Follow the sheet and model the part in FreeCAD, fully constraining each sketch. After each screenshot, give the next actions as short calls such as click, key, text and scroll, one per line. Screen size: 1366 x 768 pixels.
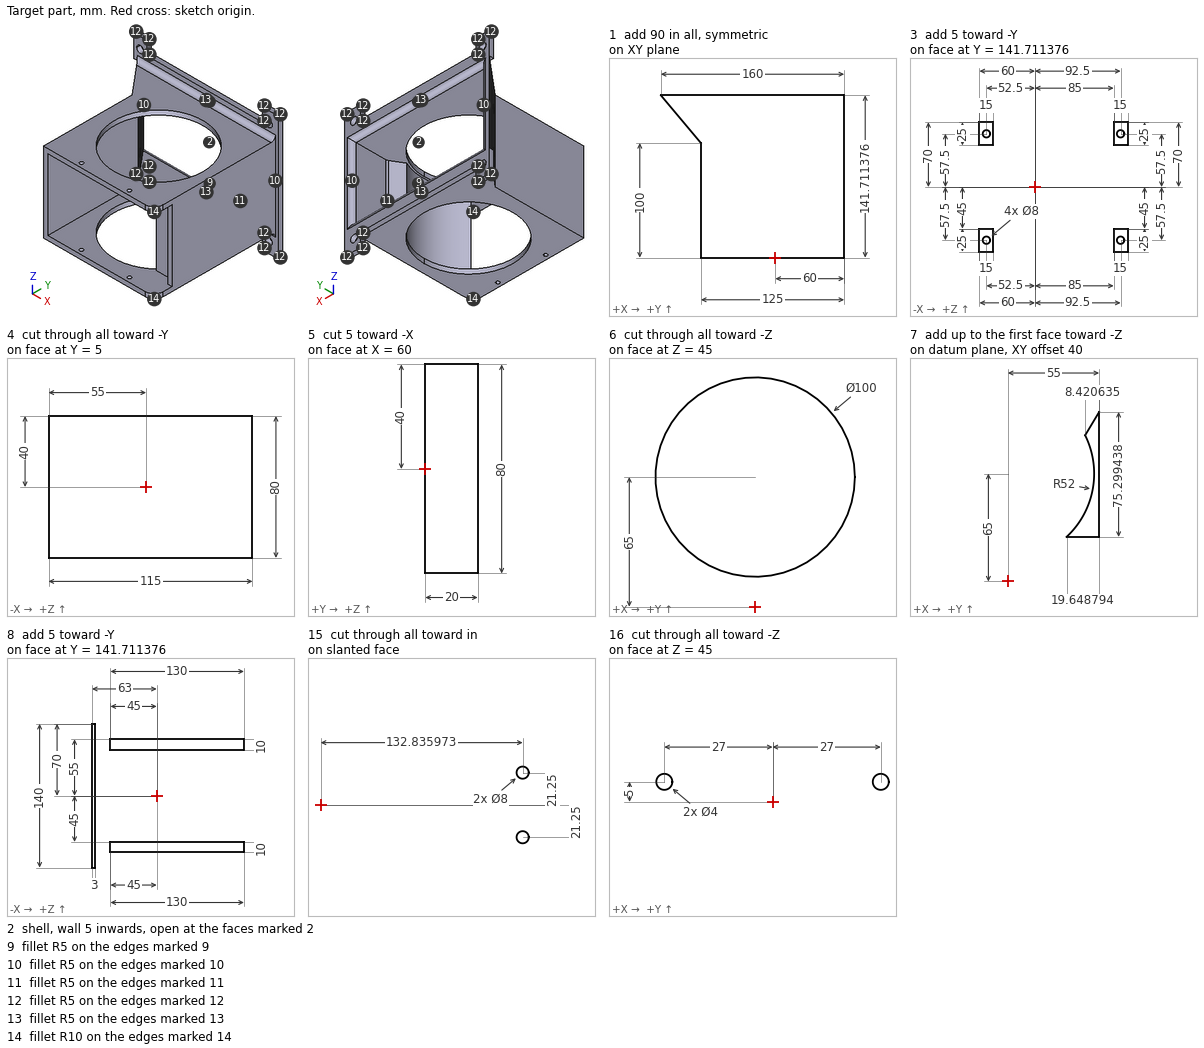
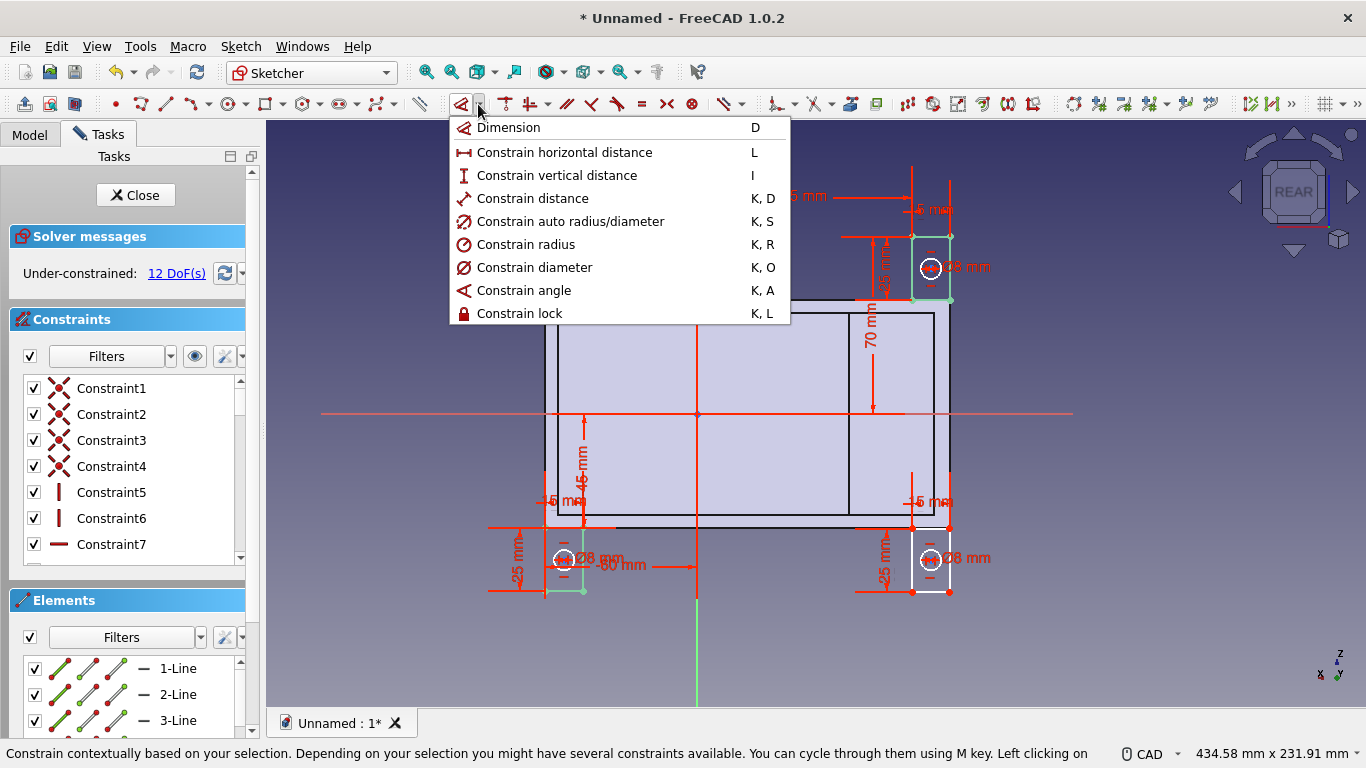
click(620, 152)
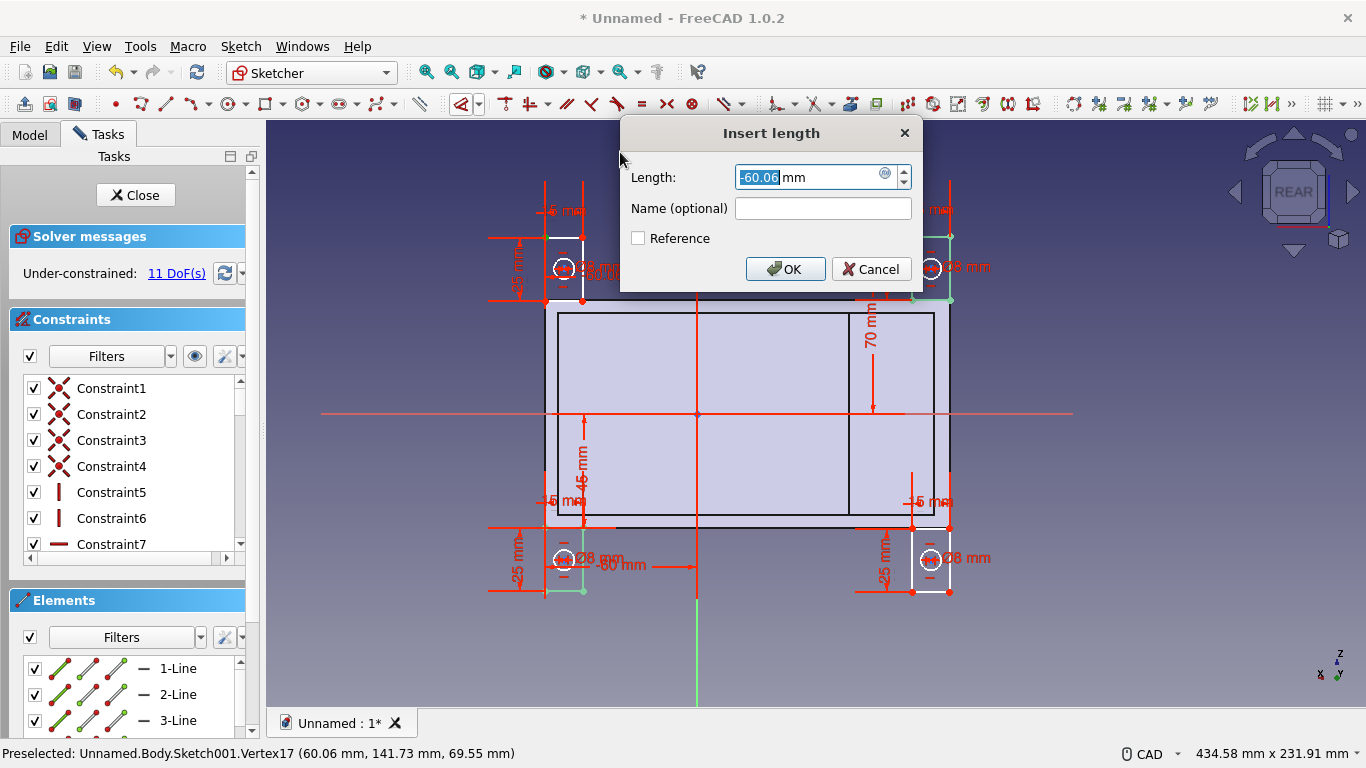
text(-60)
key(Return)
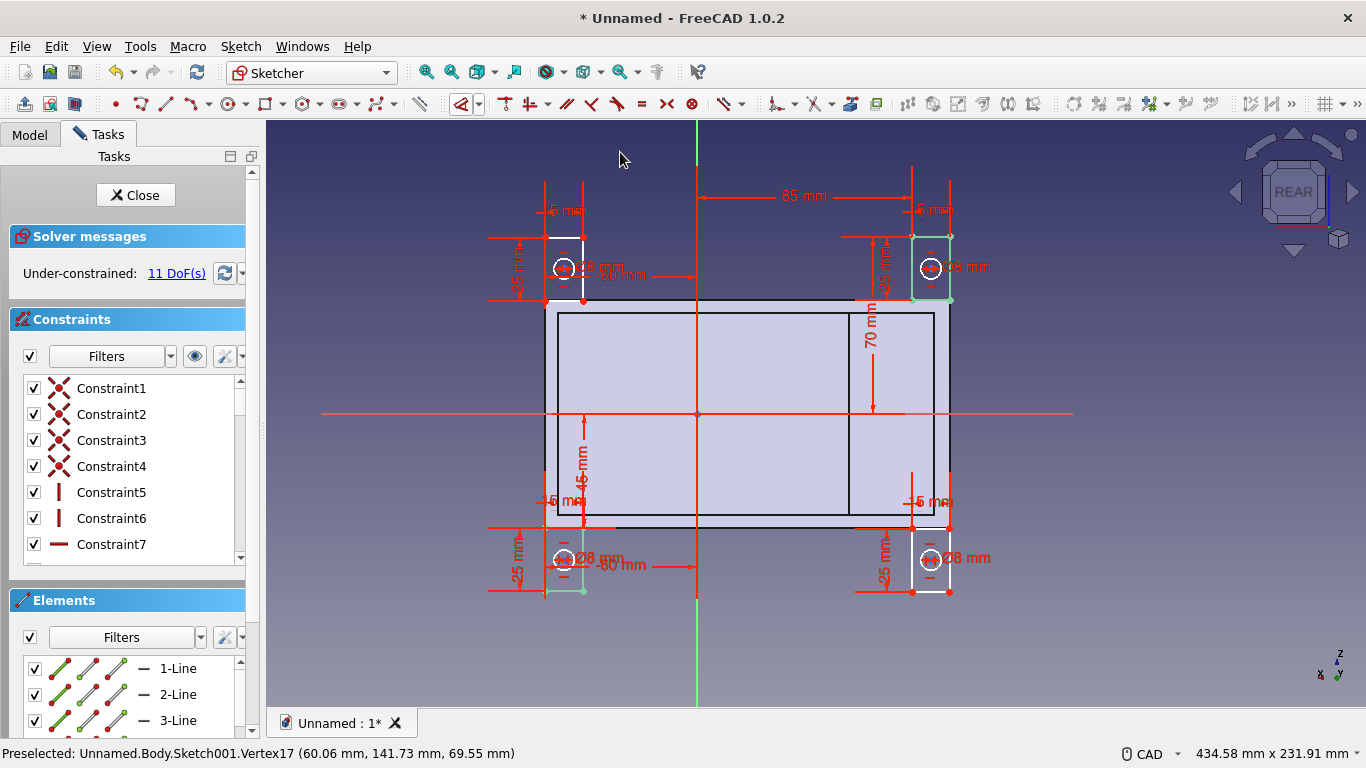
click(545, 238)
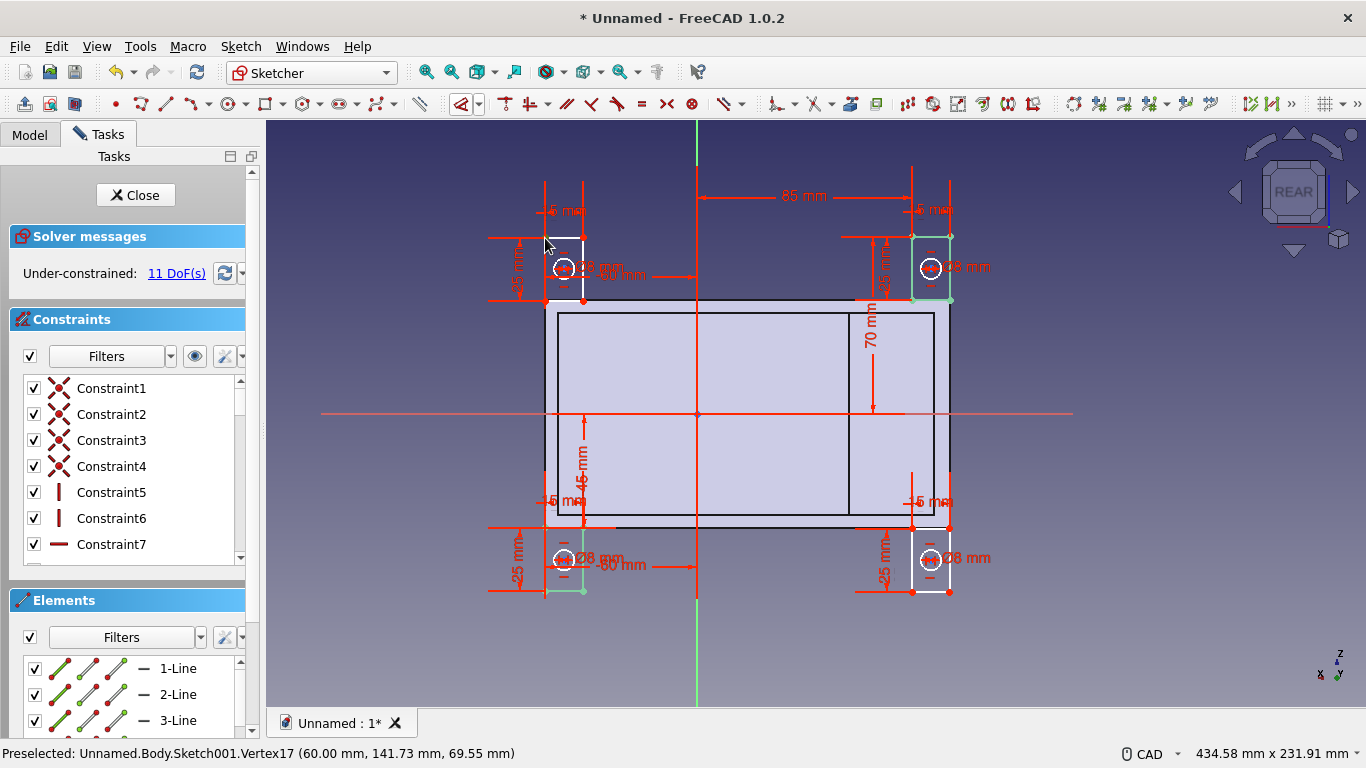
click(478, 104)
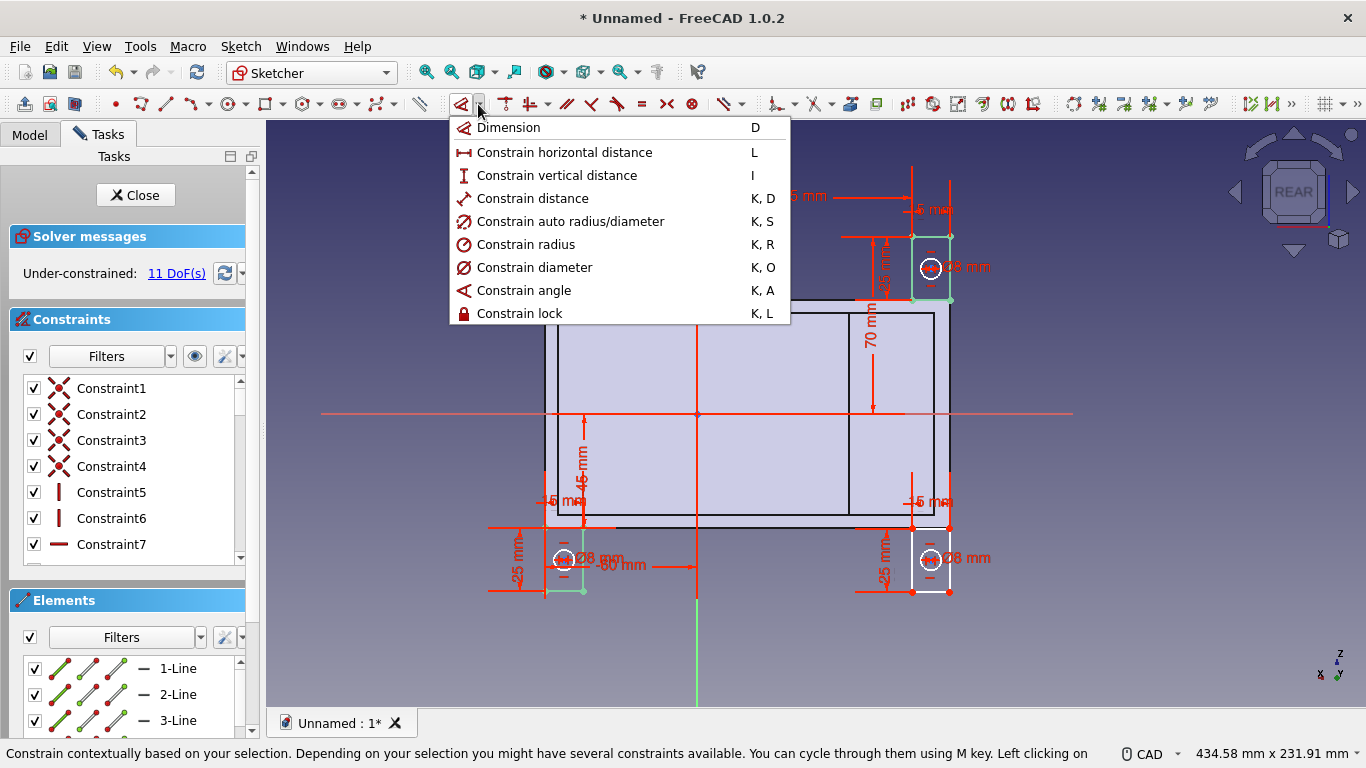
click(620, 176)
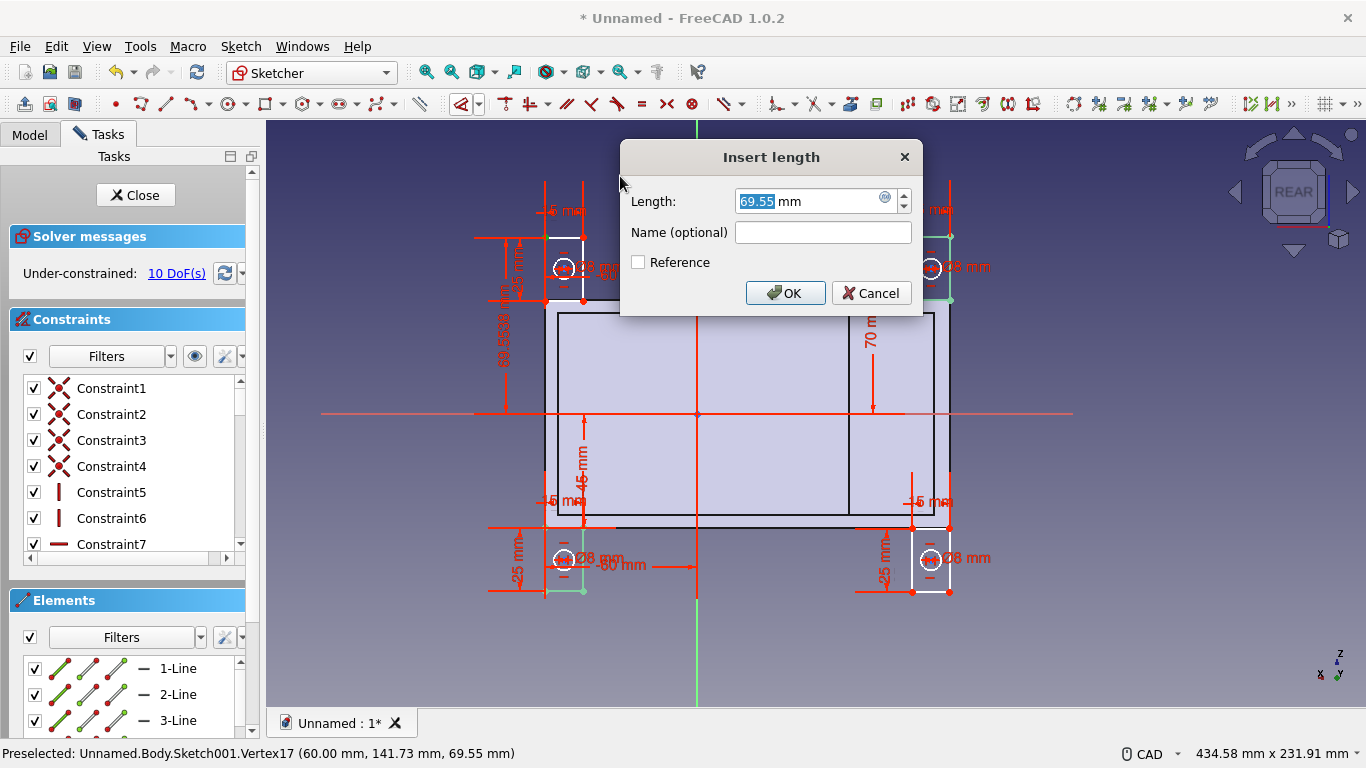
text(70)
key(Return)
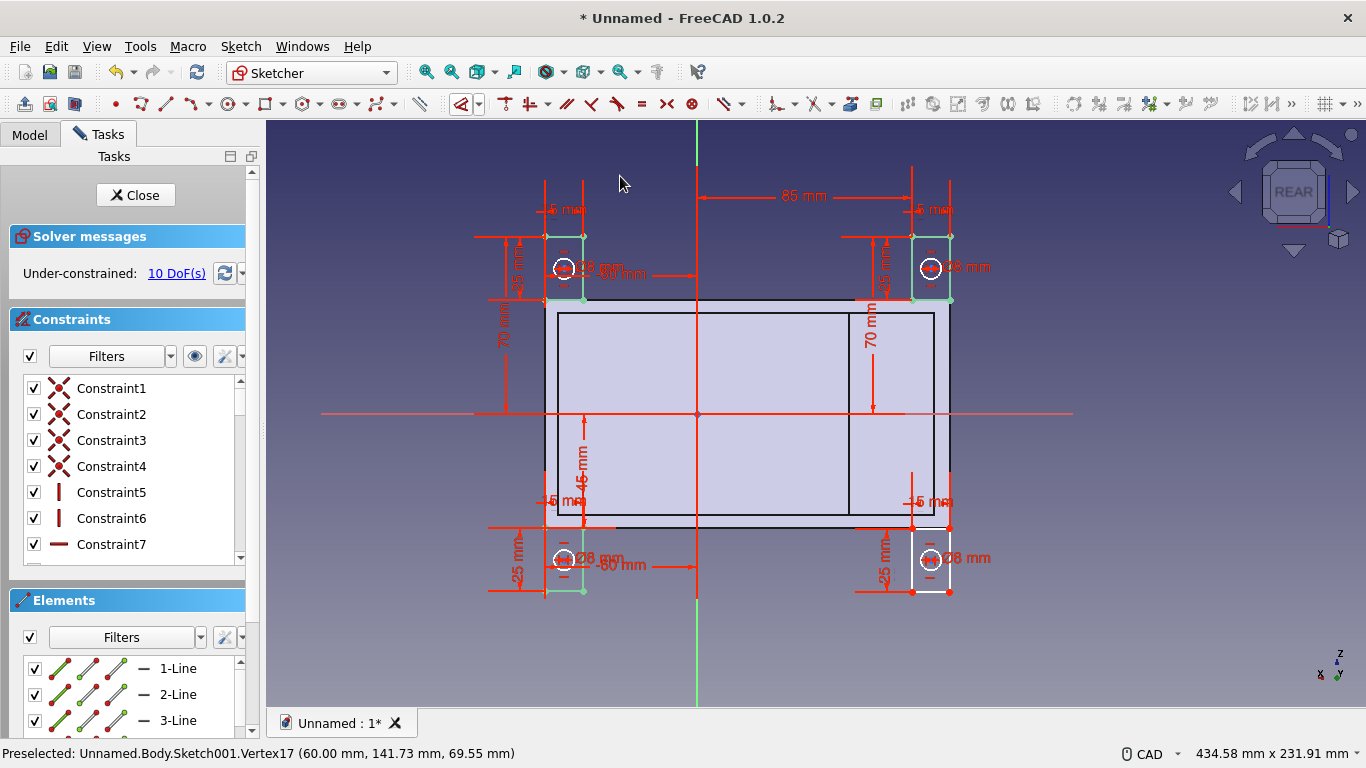
click(912, 529)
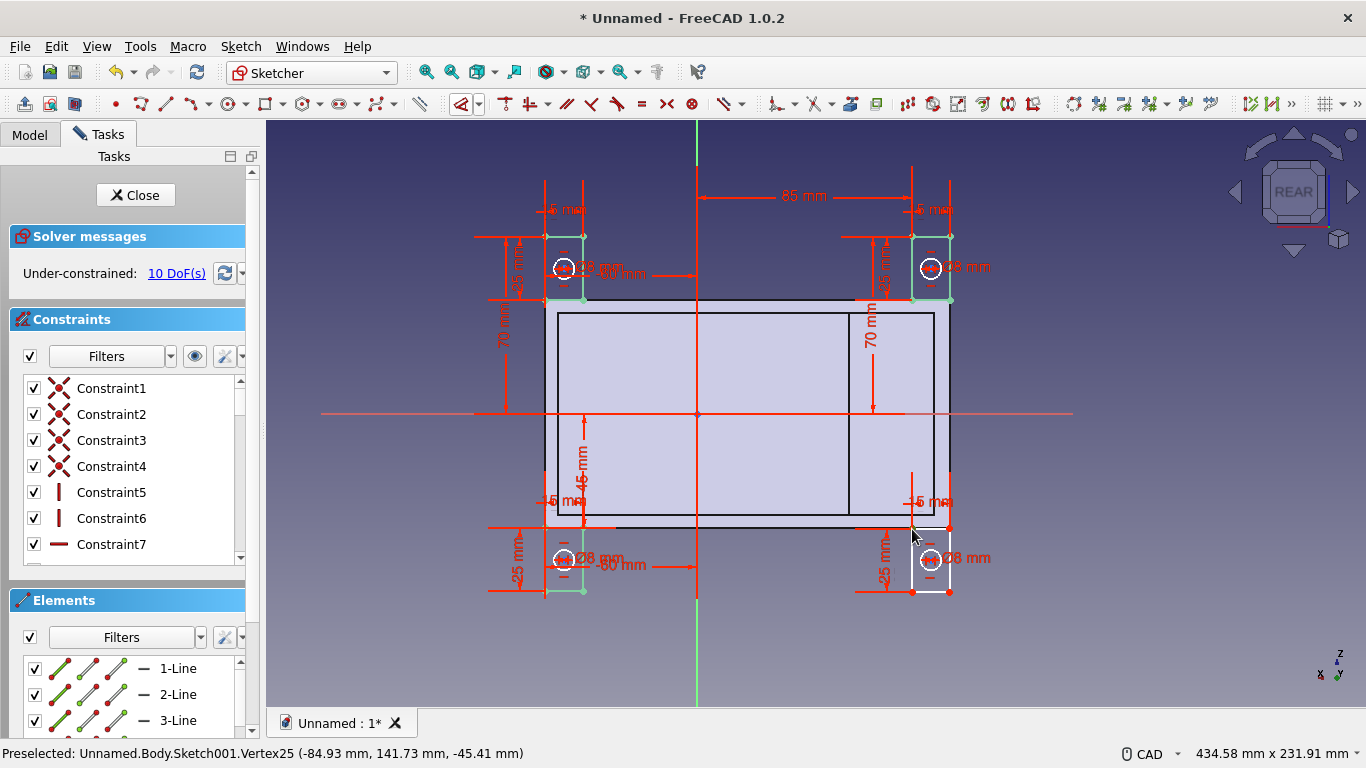
key(l)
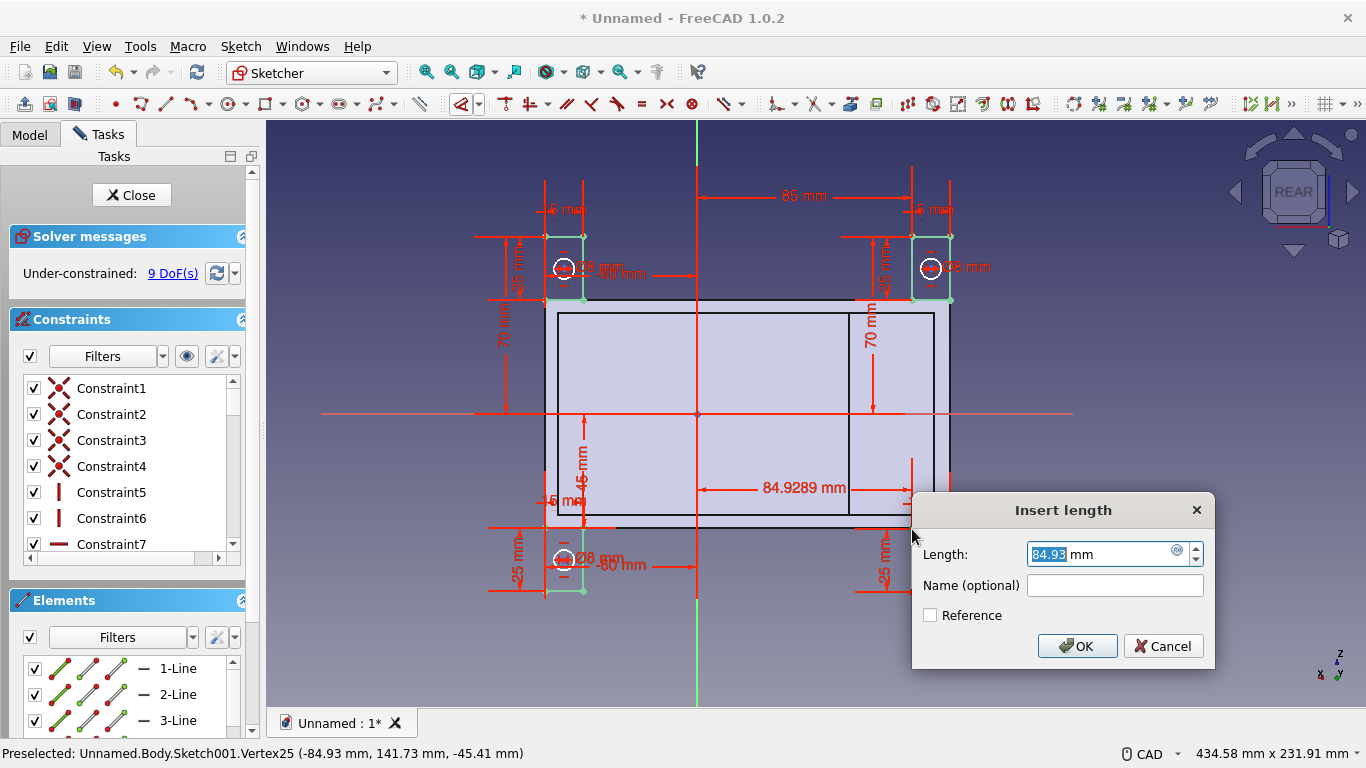
text(85)
key(Return)